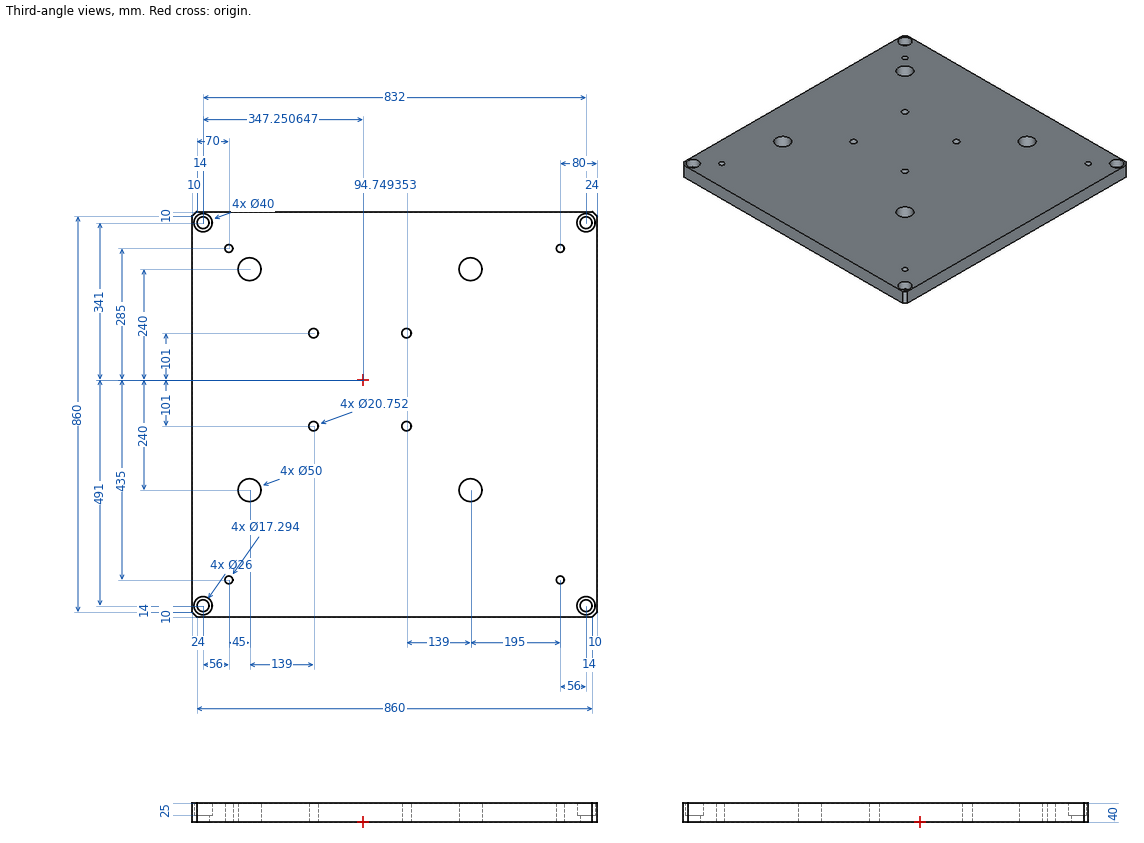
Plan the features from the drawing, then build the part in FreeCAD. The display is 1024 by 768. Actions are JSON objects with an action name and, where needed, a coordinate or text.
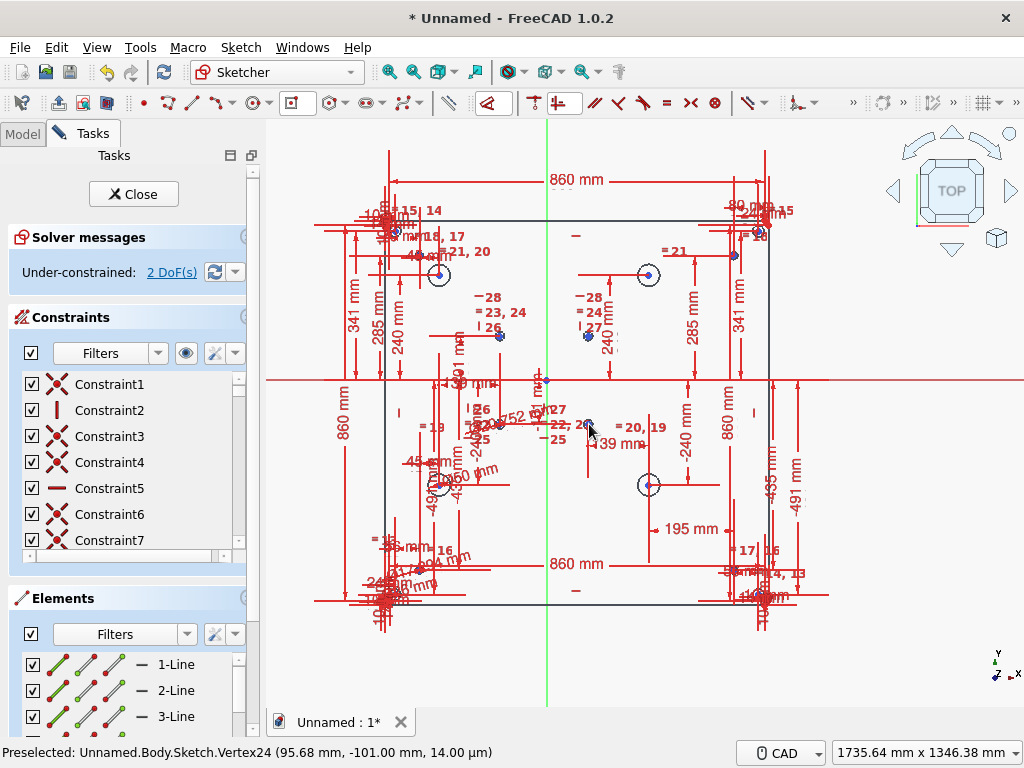
{"action": "left_click", "coordinate": [588, 336]}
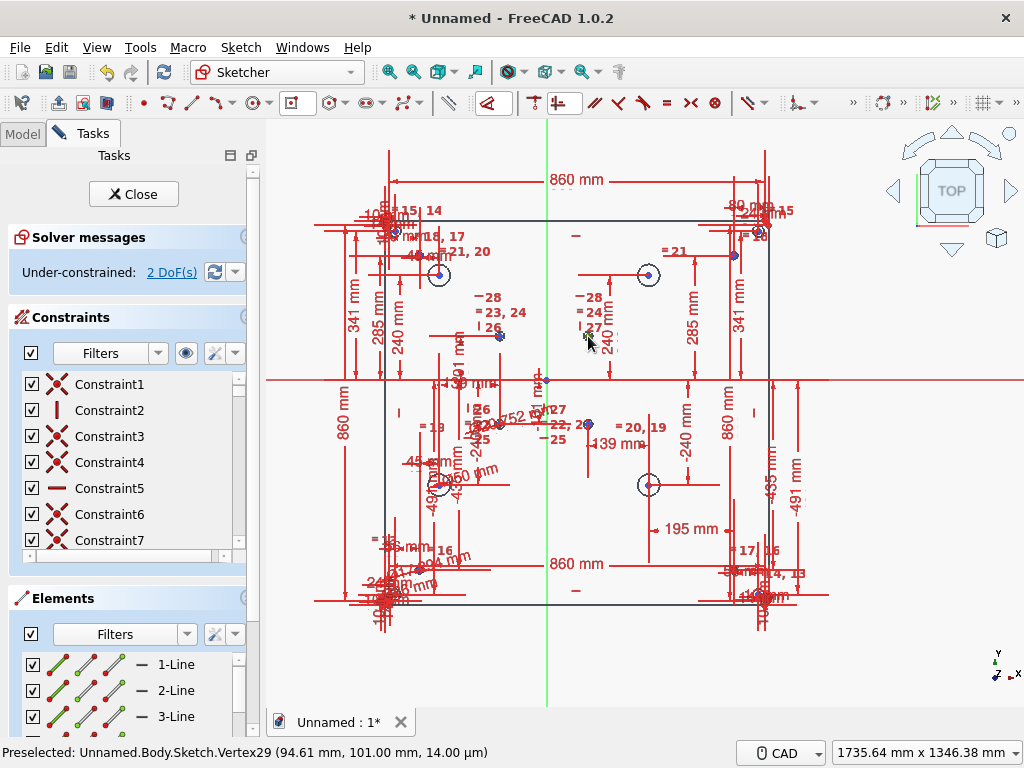
{"action": "left_click", "coordinate": [649, 275]}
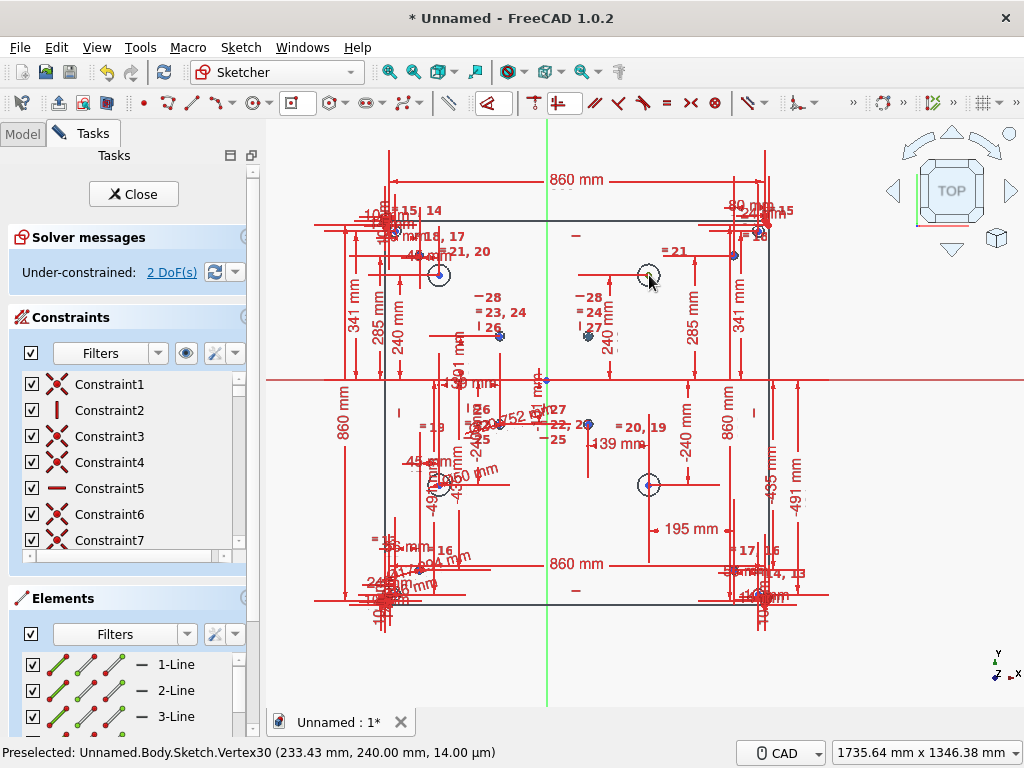
{"action": "key", "text": "l"}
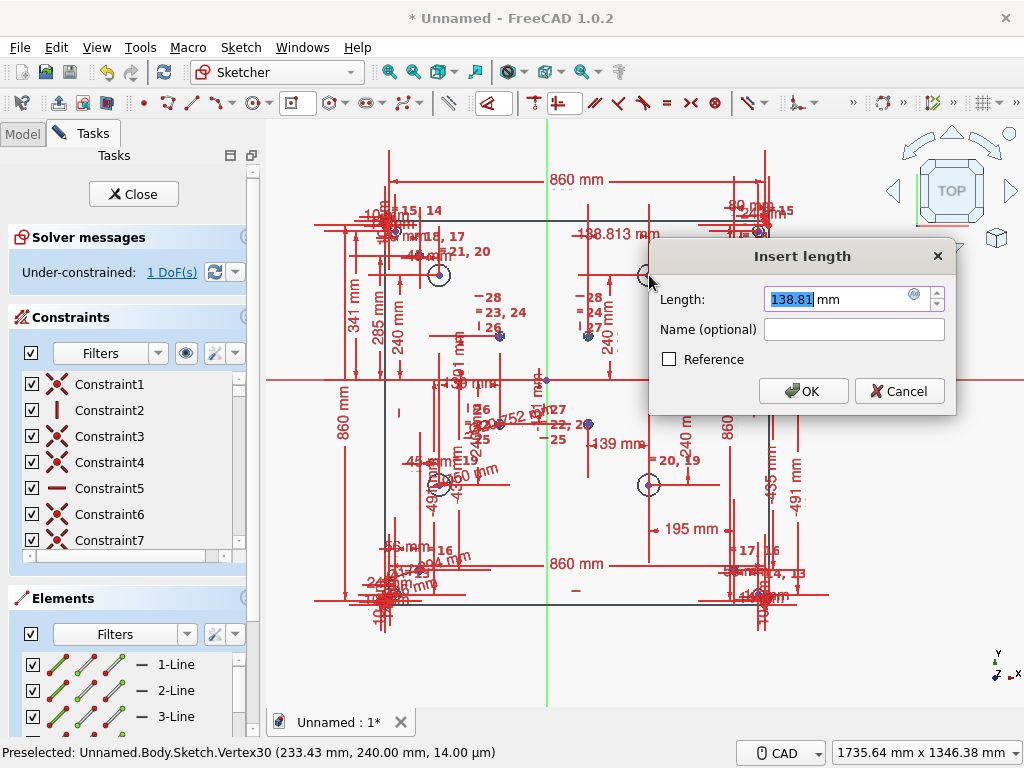
{"action": "type", "text": "139"}
{"action": "key", "text": "Return"}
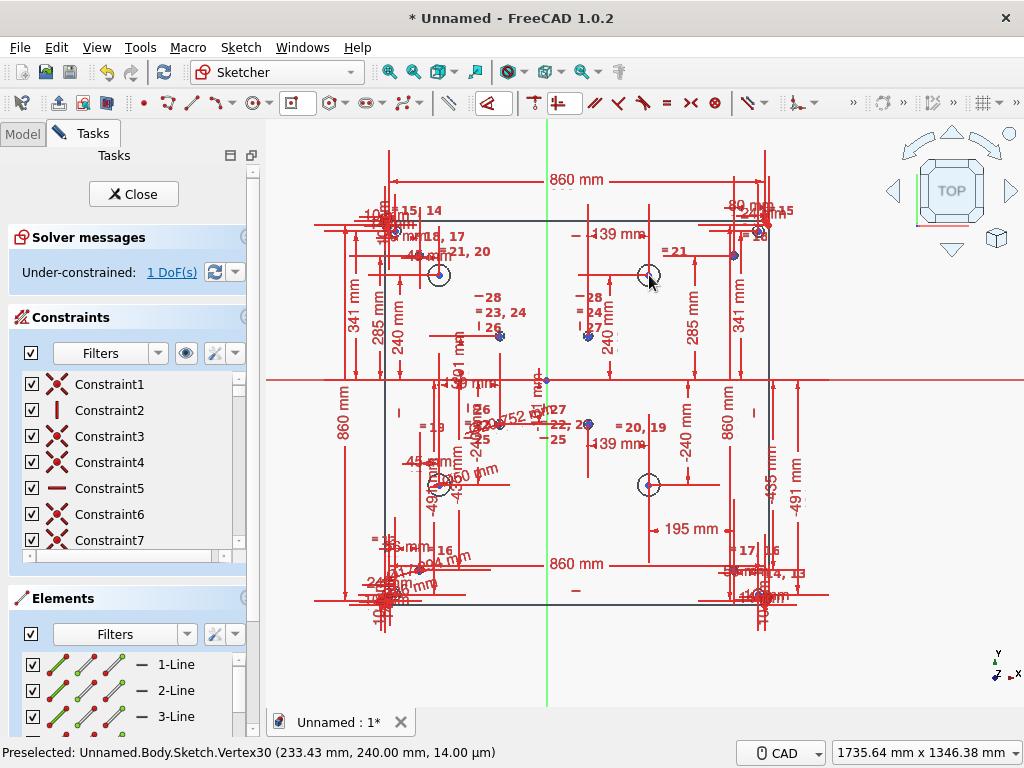
{"action": "left_click", "coordinate": [588, 424]}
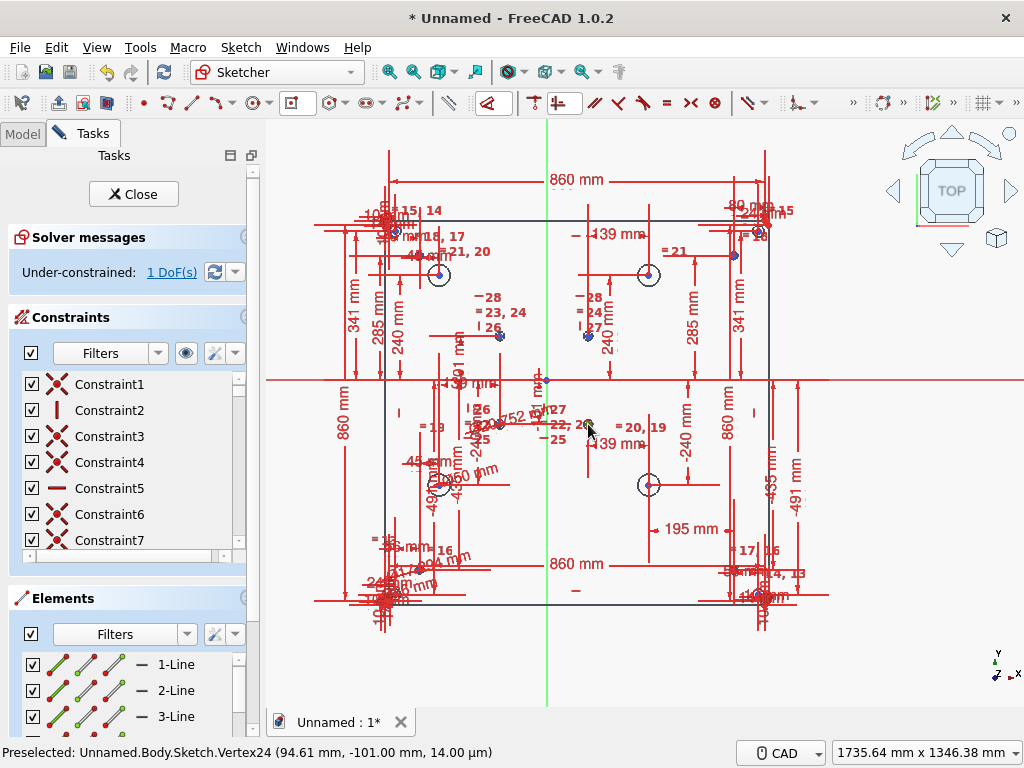
{"action": "left_click", "coordinate": [506, 104]}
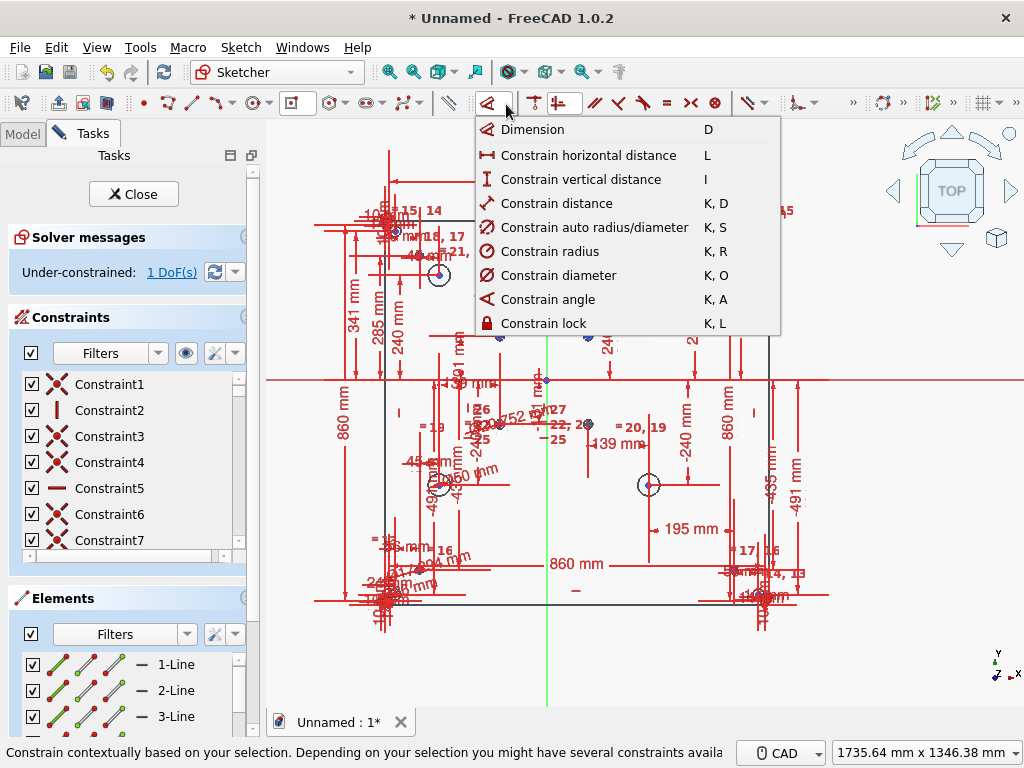
{"action": "left_click", "coordinate": [628, 155]}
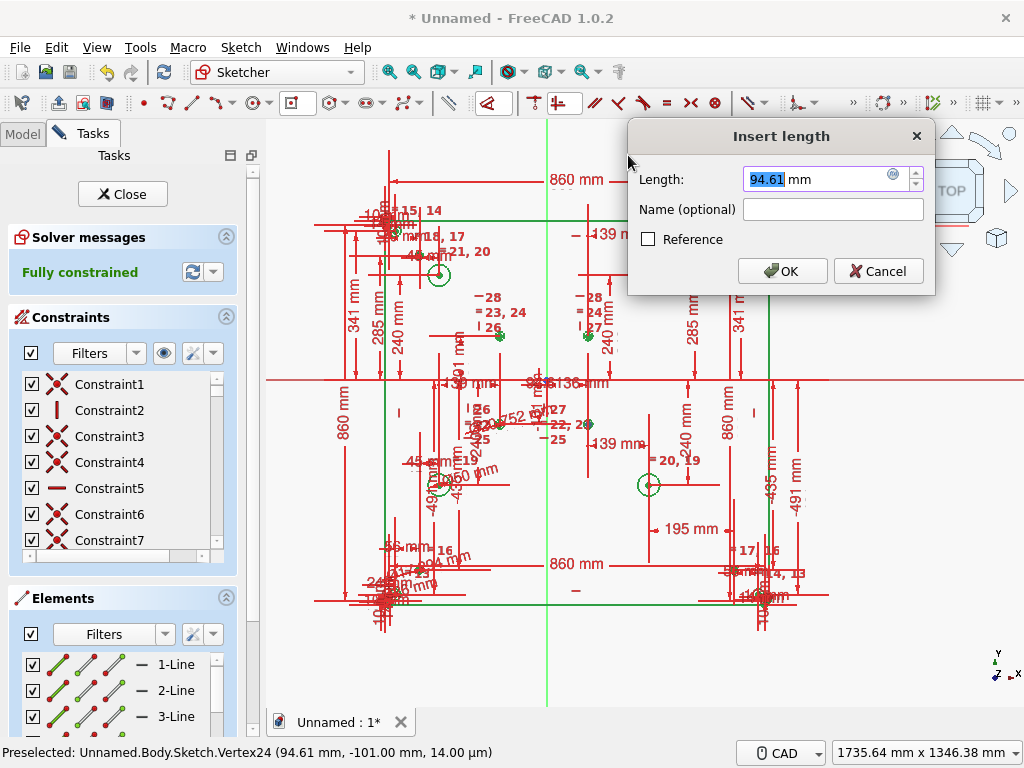
{"action": "type", "text": "94.749353"}
{"action": "key", "text": "Return"}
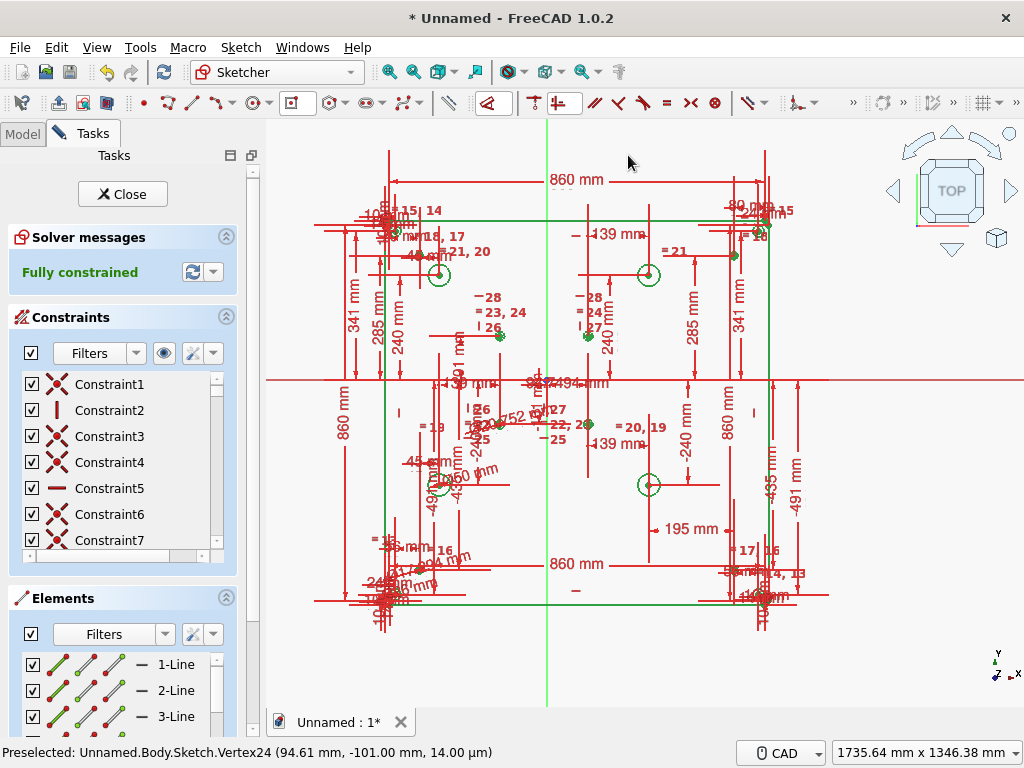
{"action": "left_click", "coordinate": [123, 194]}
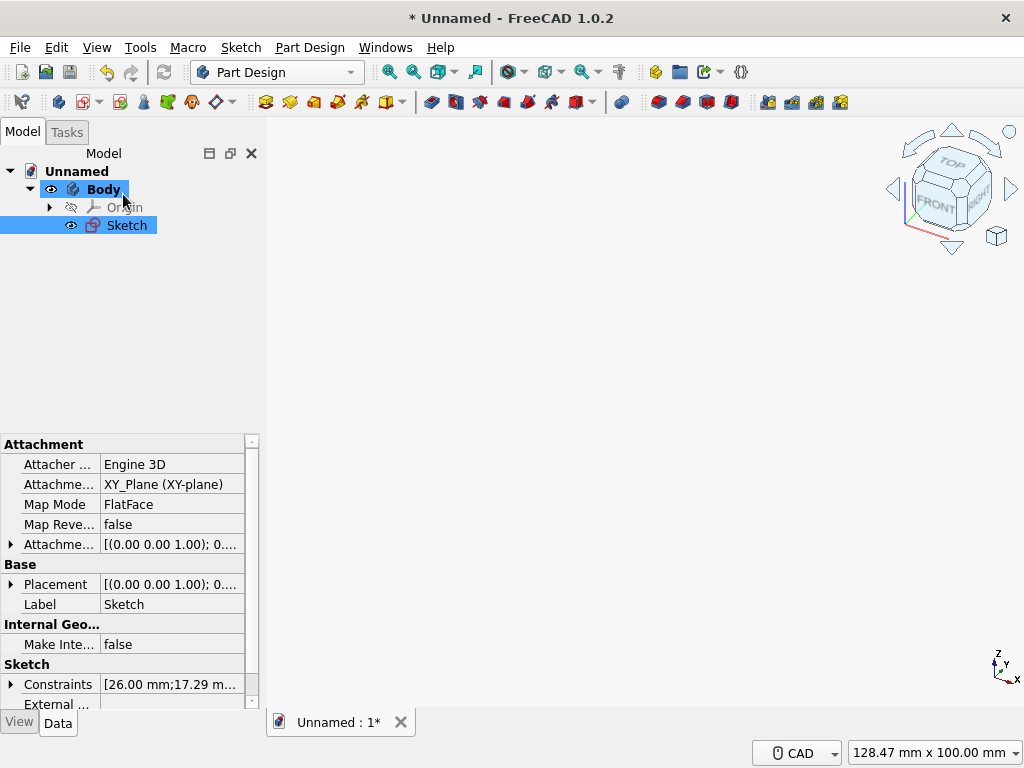
{"action": "left_click", "coordinate": [266, 102]}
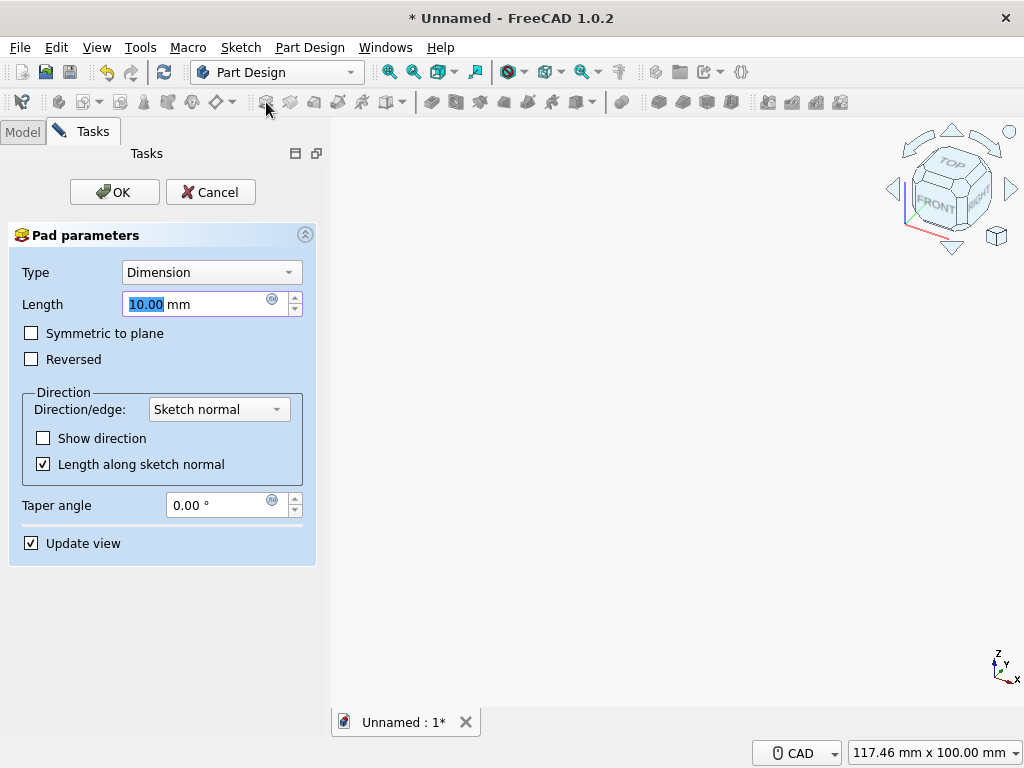
{"action": "type", "text": "40"}
{"action": "key", "text": "Tab"}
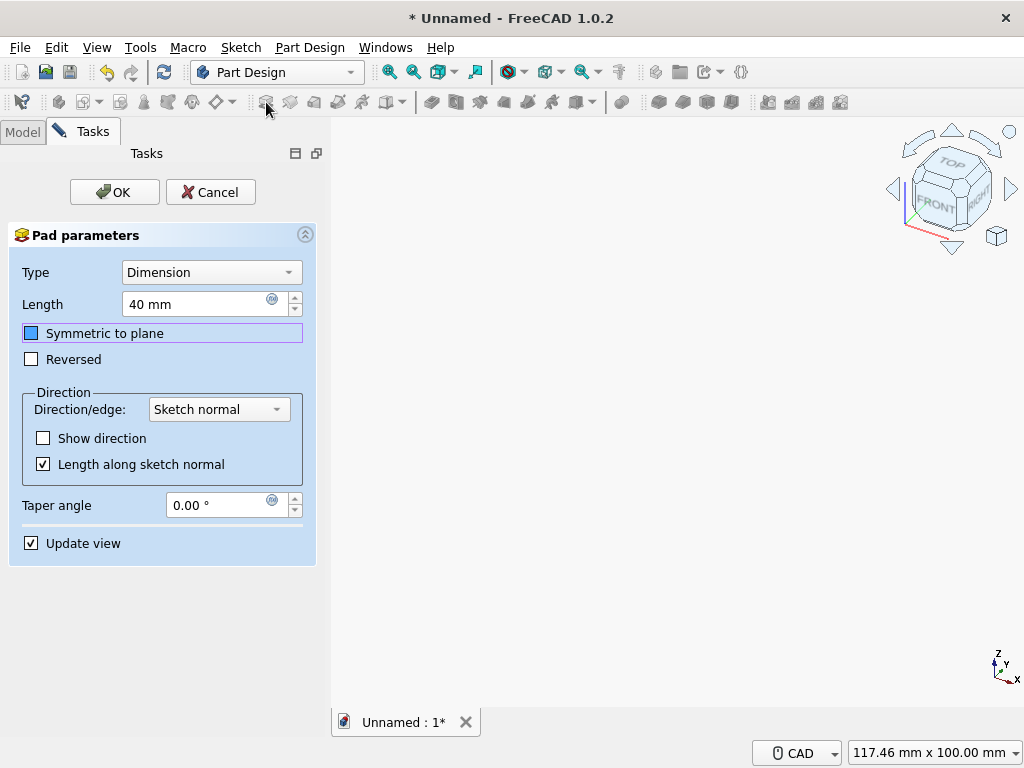
{"action": "left_click", "coordinate": [115, 192]}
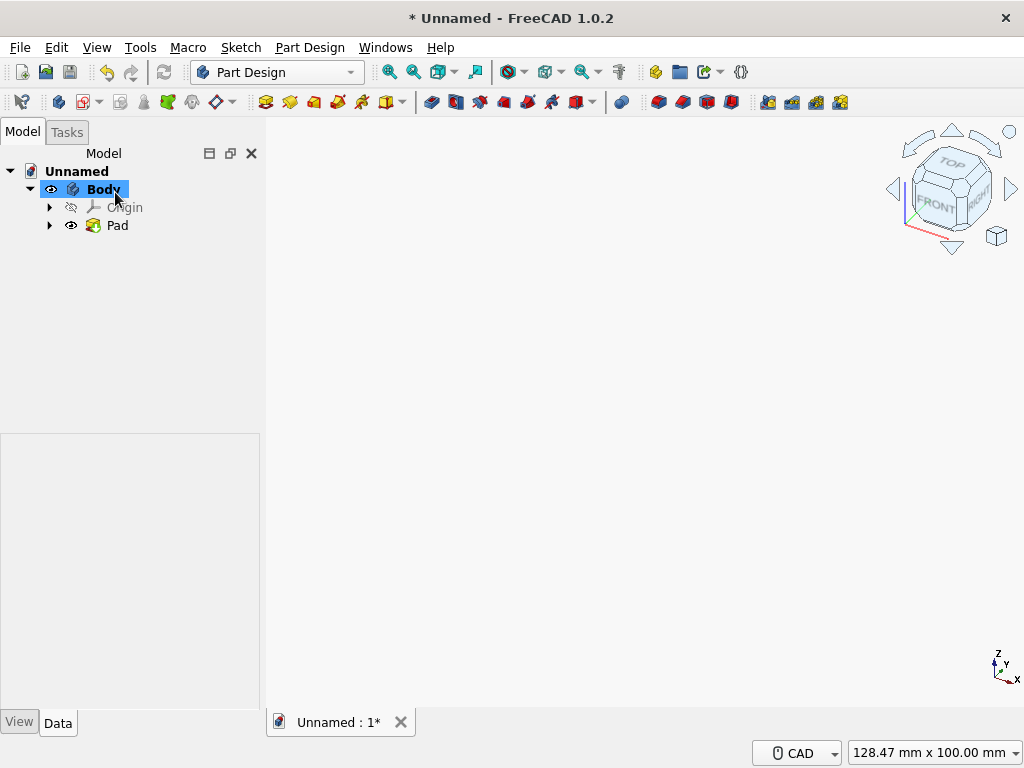
{"action": "left_click", "coordinate": [390, 72]}